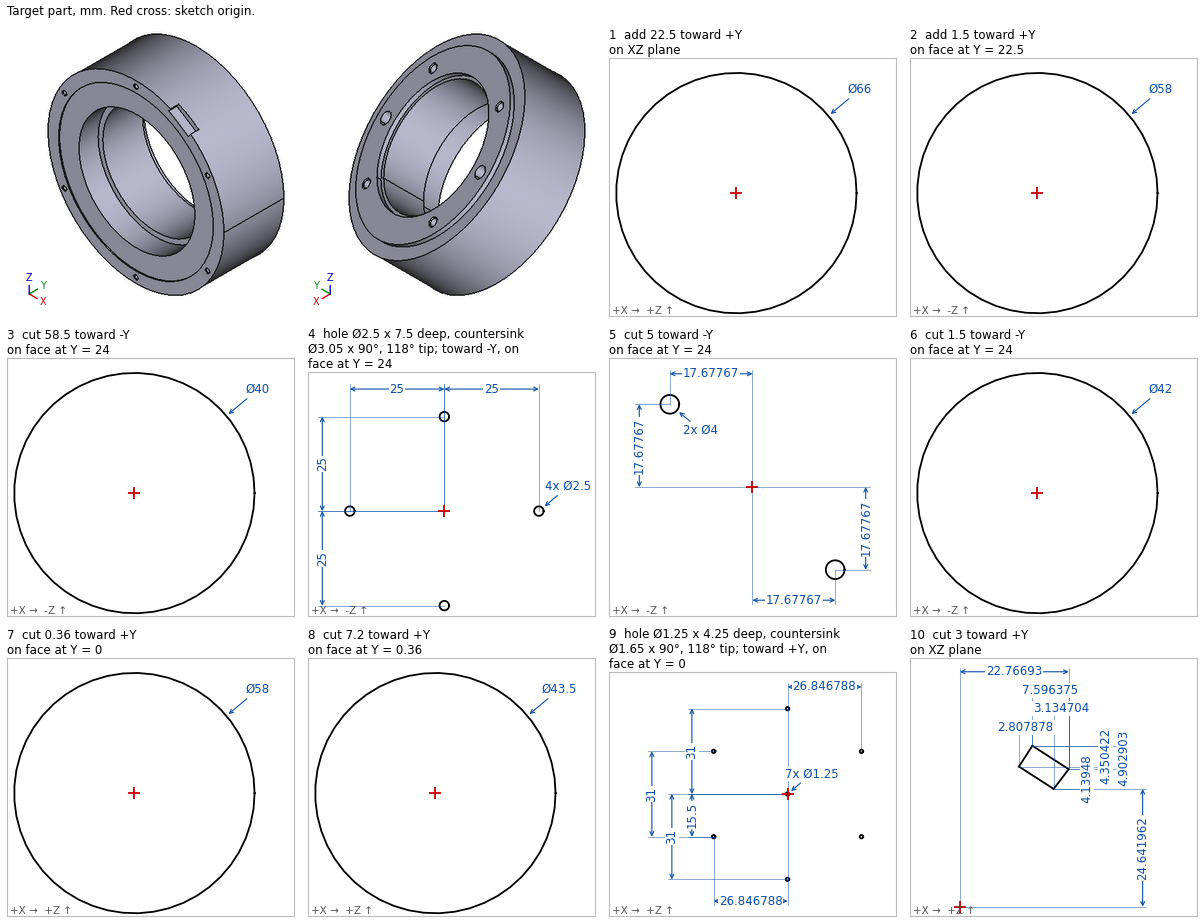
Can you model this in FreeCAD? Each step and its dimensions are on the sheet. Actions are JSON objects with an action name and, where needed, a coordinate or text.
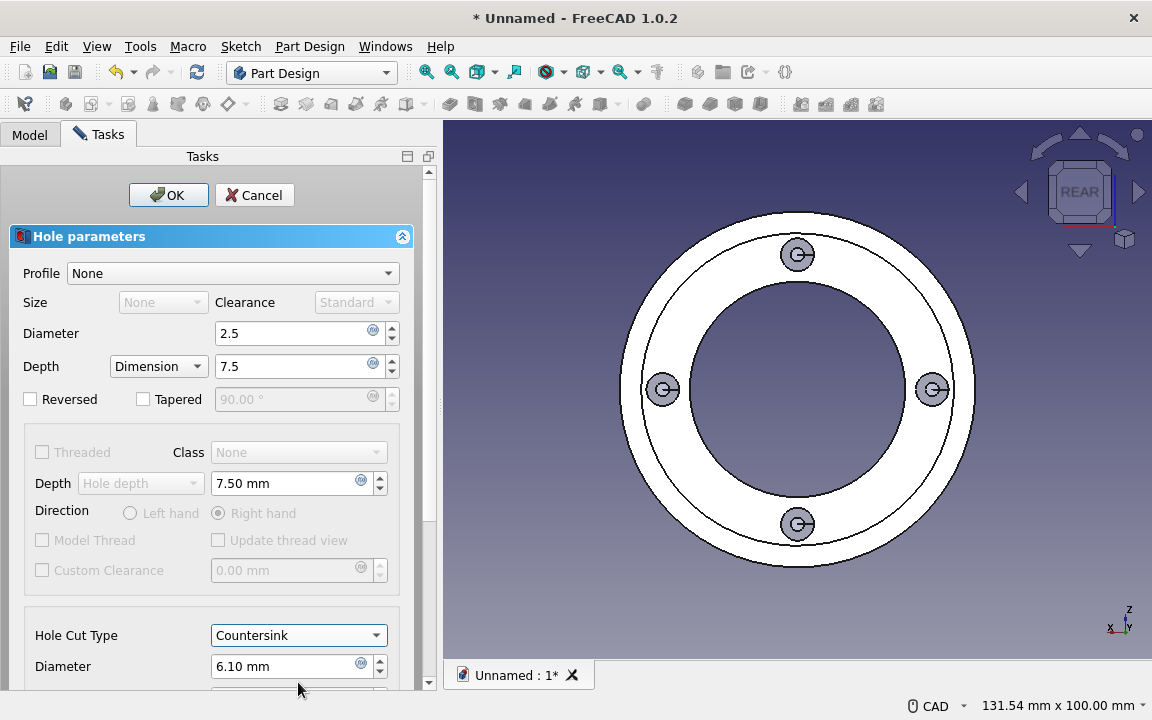
{"action": "triple_click", "coordinate": [292, 666]}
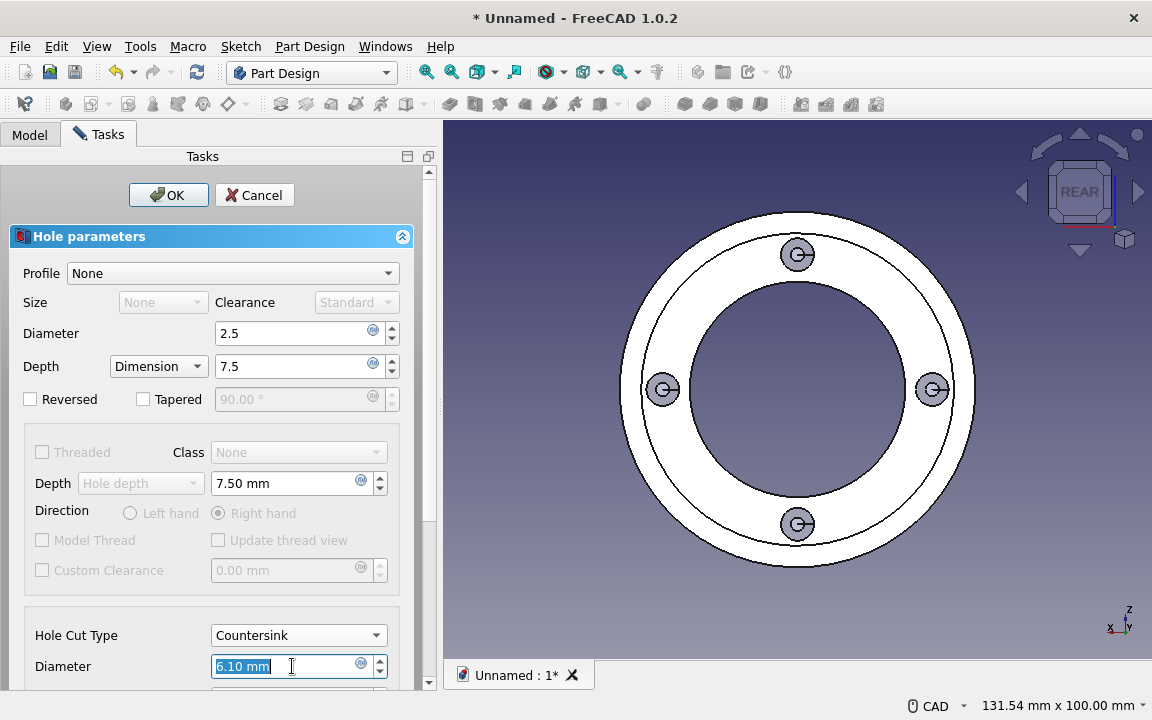
{"action": "type", "text": "3.05"}
{"action": "key", "text": "Tab"}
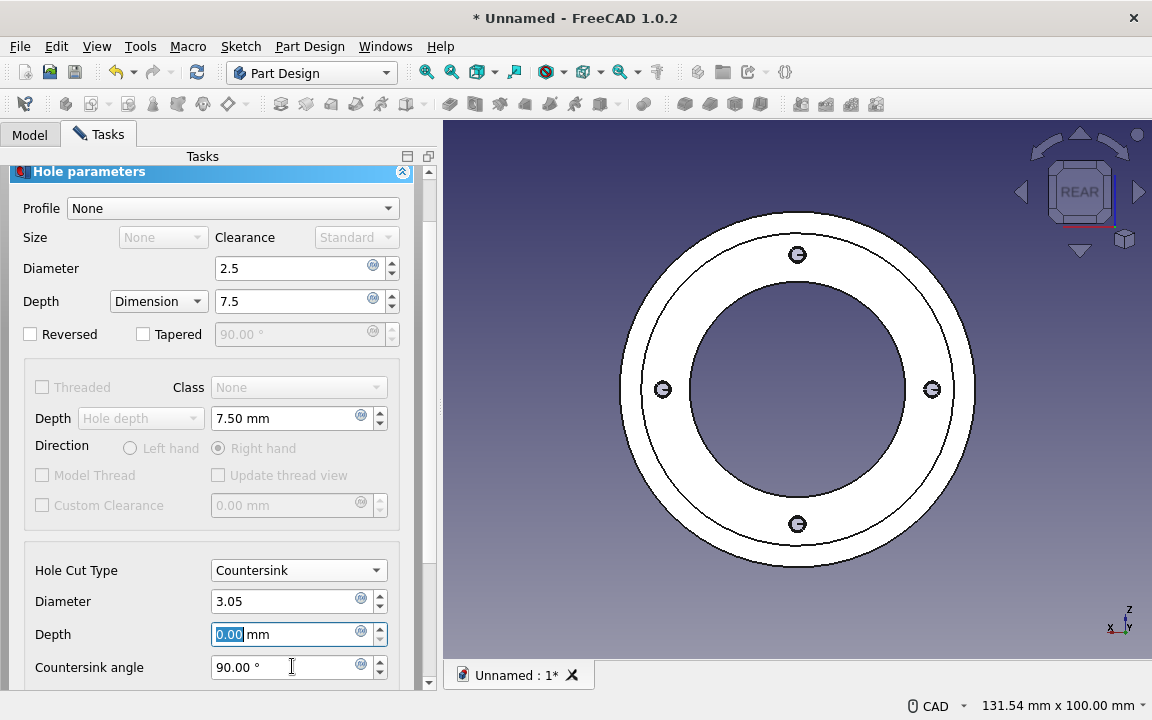
{"action": "scroll", "coordinate": [429, 428], "scroll_direction": "up", "scroll_amount": 2}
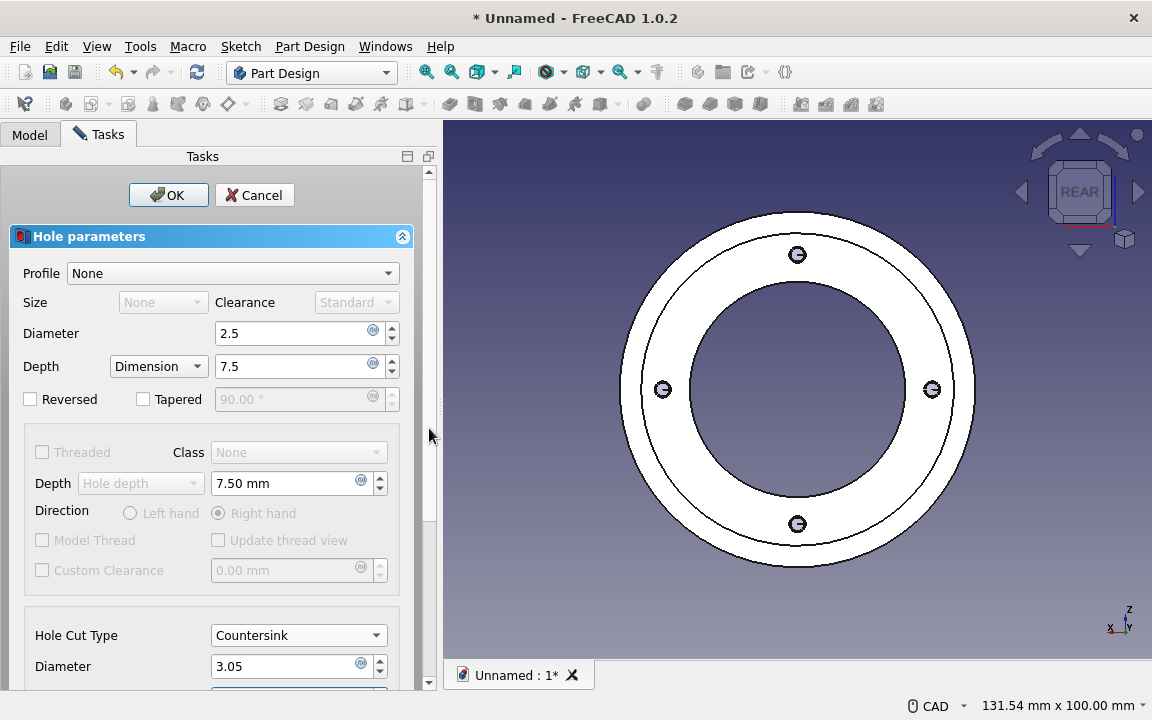
{"action": "left_click", "coordinate": [169, 195]}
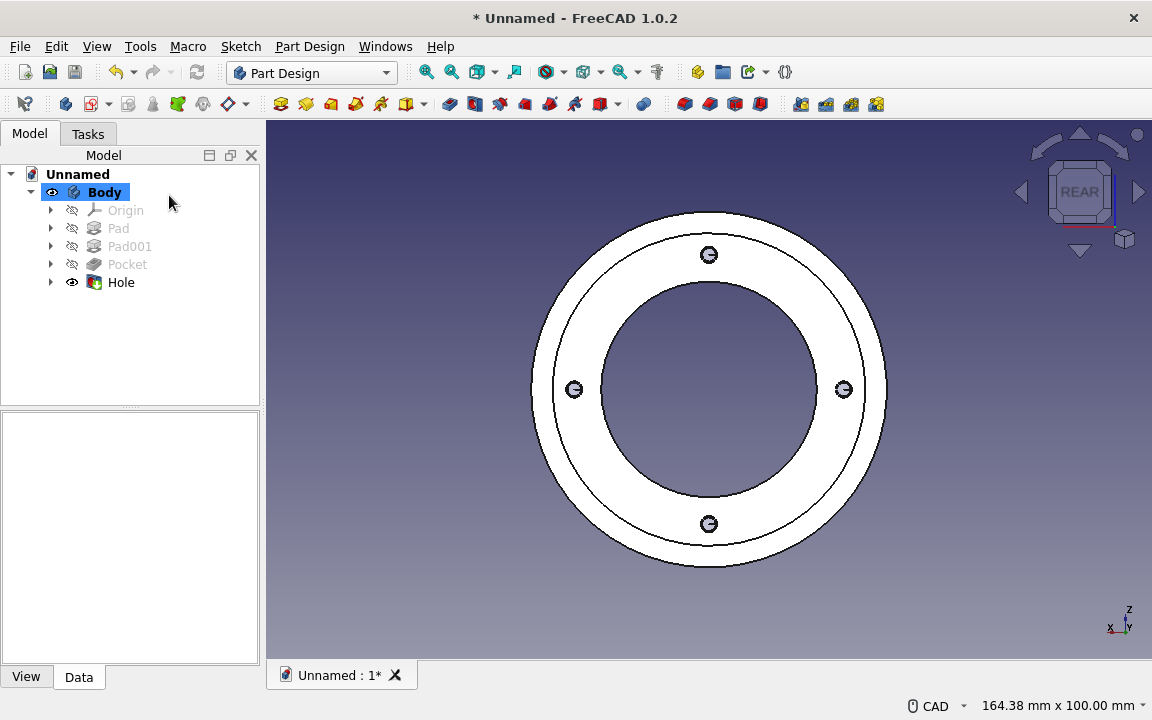
{"action": "left_click", "coordinate": [620, 478]}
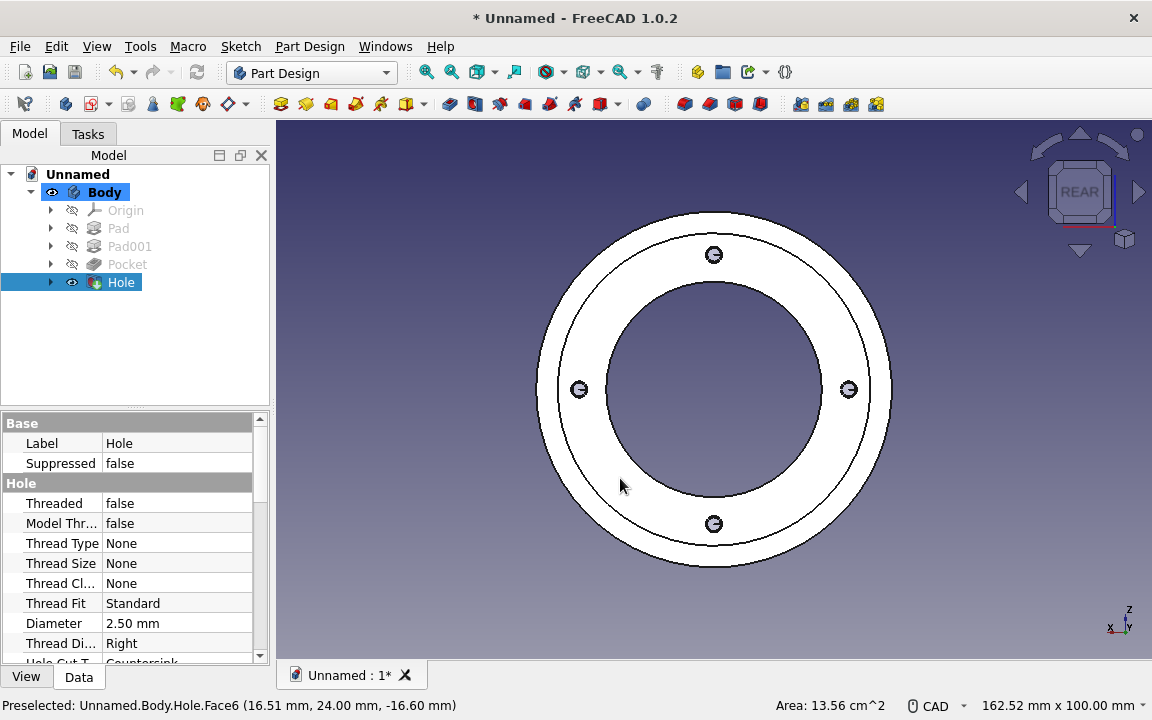
{"action": "left_click", "coordinate": [90, 104]}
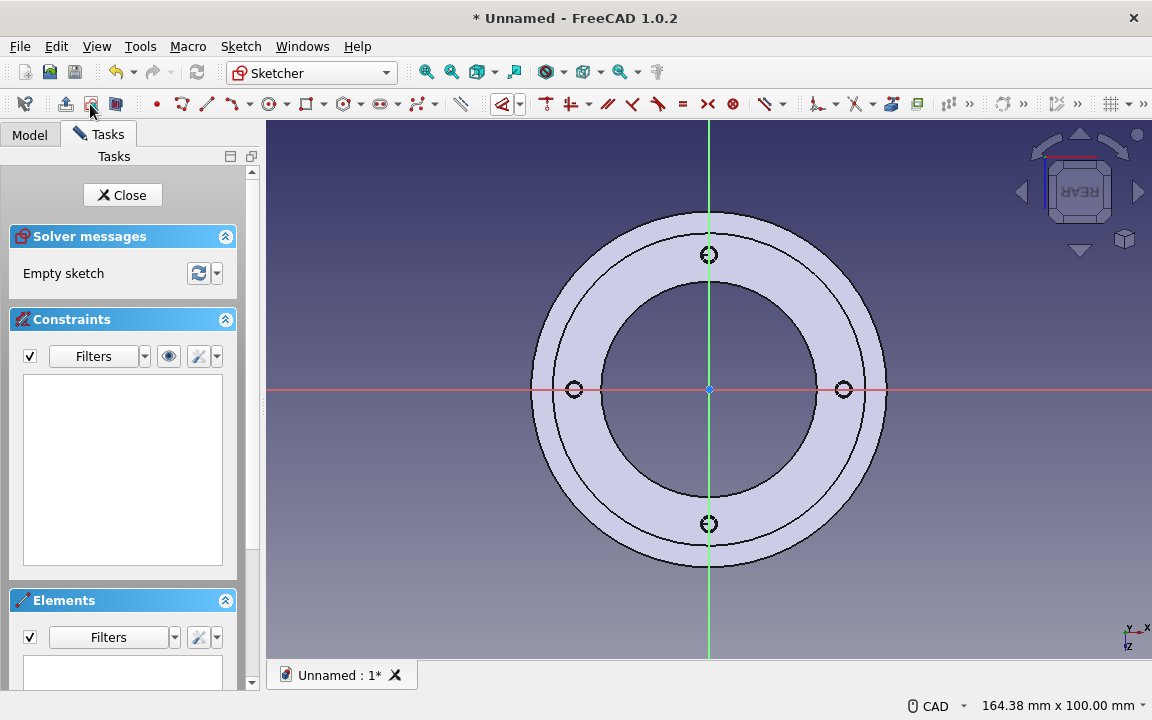
{"action": "scroll", "coordinate": [848, 389], "scroll_direction": "up", "scroll_amount": 2}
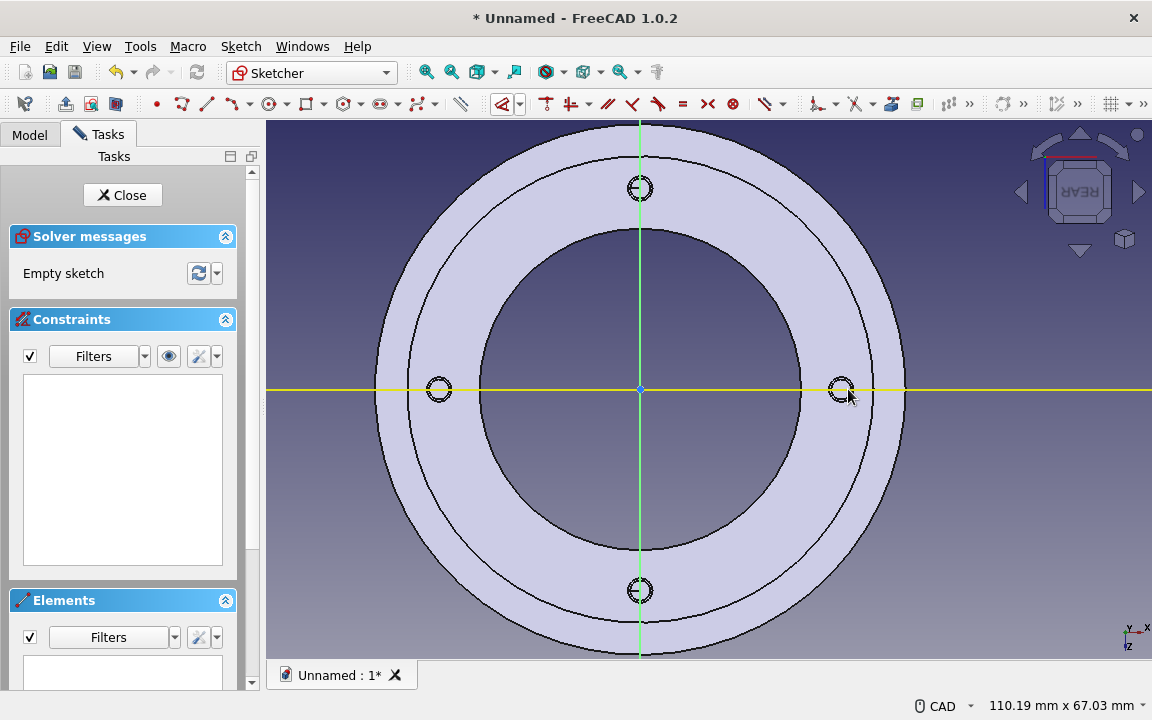
{"action": "left_click", "coordinate": [268, 104]}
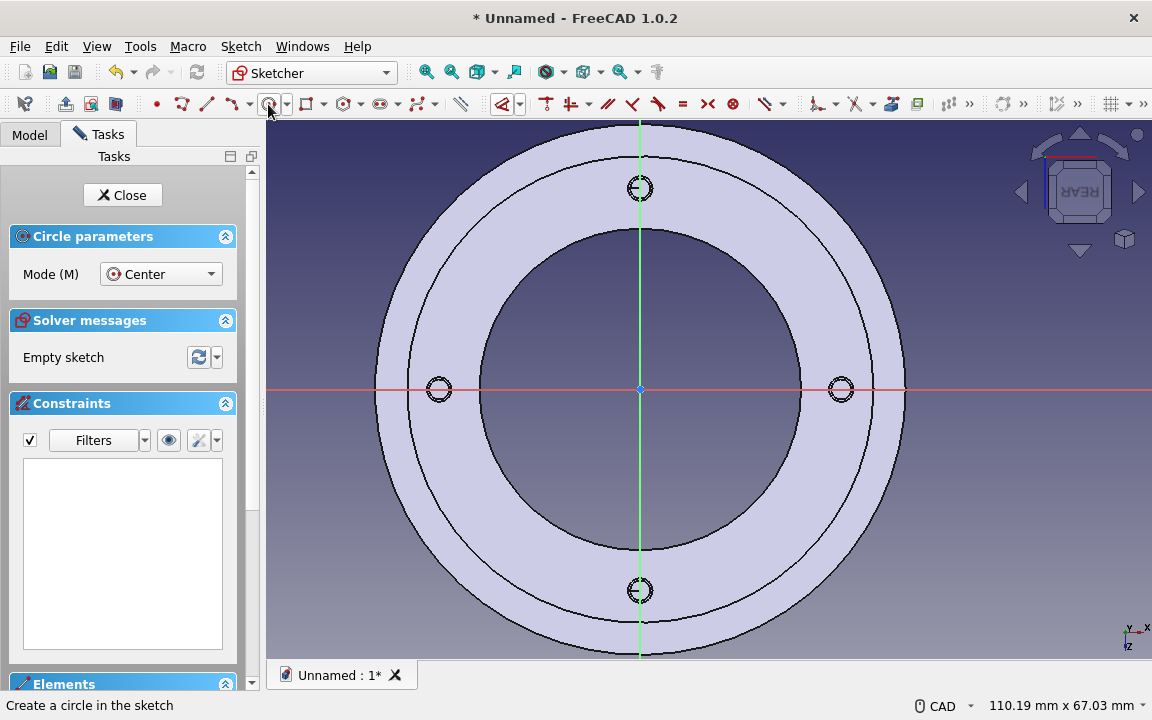
{"action": "scroll", "coordinate": [498, 247], "scroll_direction": "up", "scroll_amount": 2}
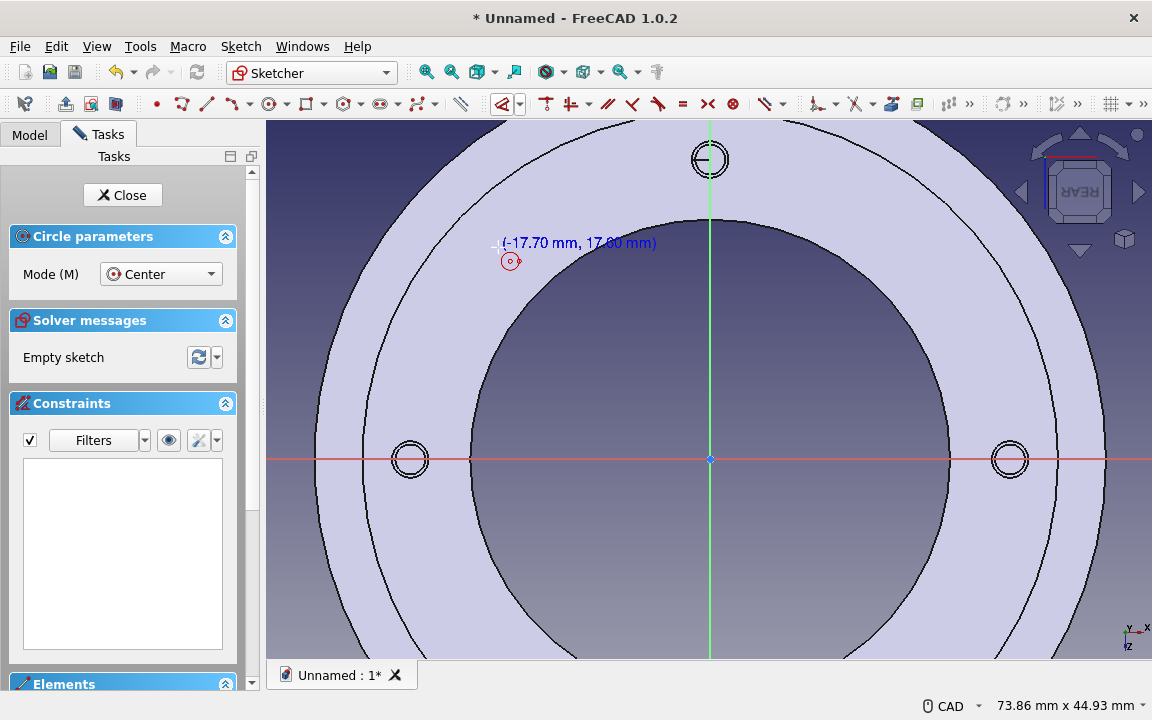
{"action": "left_click", "coordinate": [498, 247]}
{"action": "left_click", "coordinate": [515, 230]}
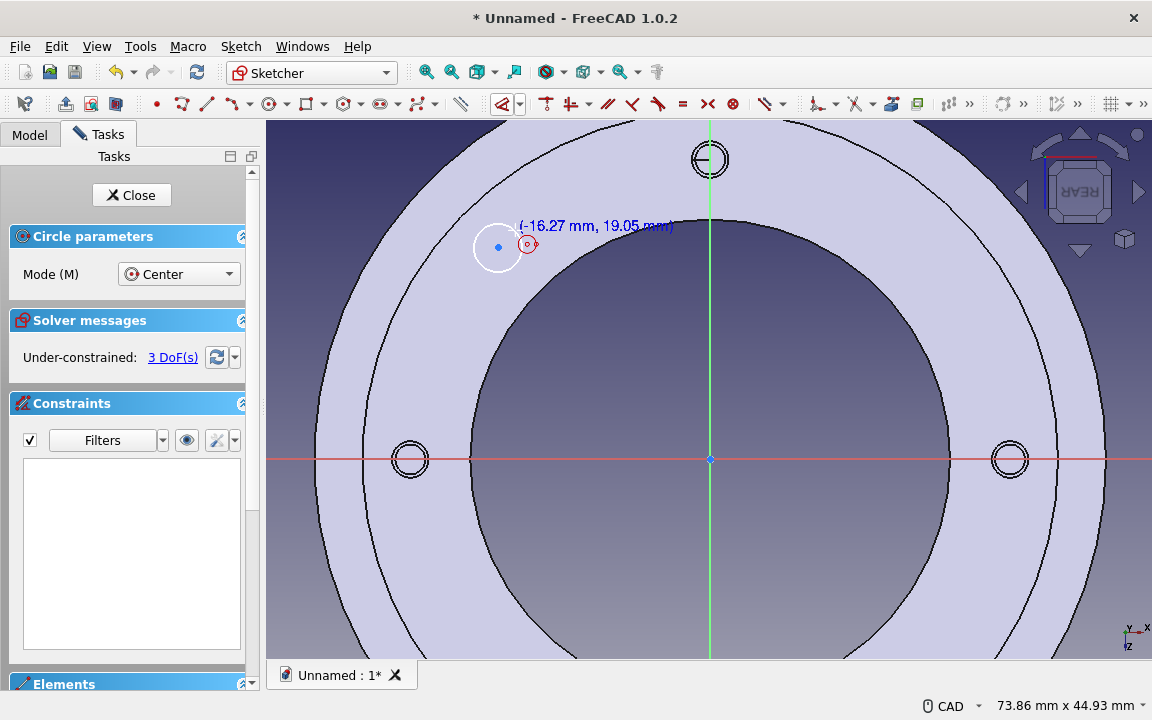
{"action": "scroll", "coordinate": [499, 247], "scroll_direction": "down", "scroll_amount": 2}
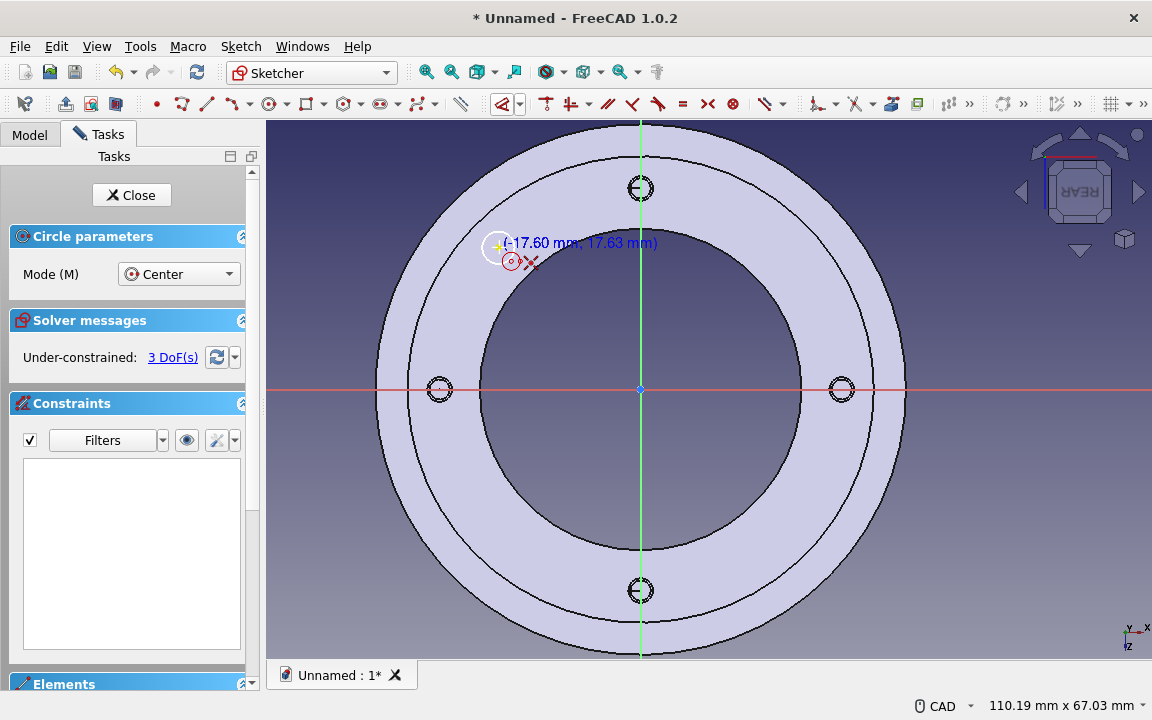
{"action": "scroll", "coordinate": [783, 532], "scroll_direction": "up", "scroll_amount": 2}